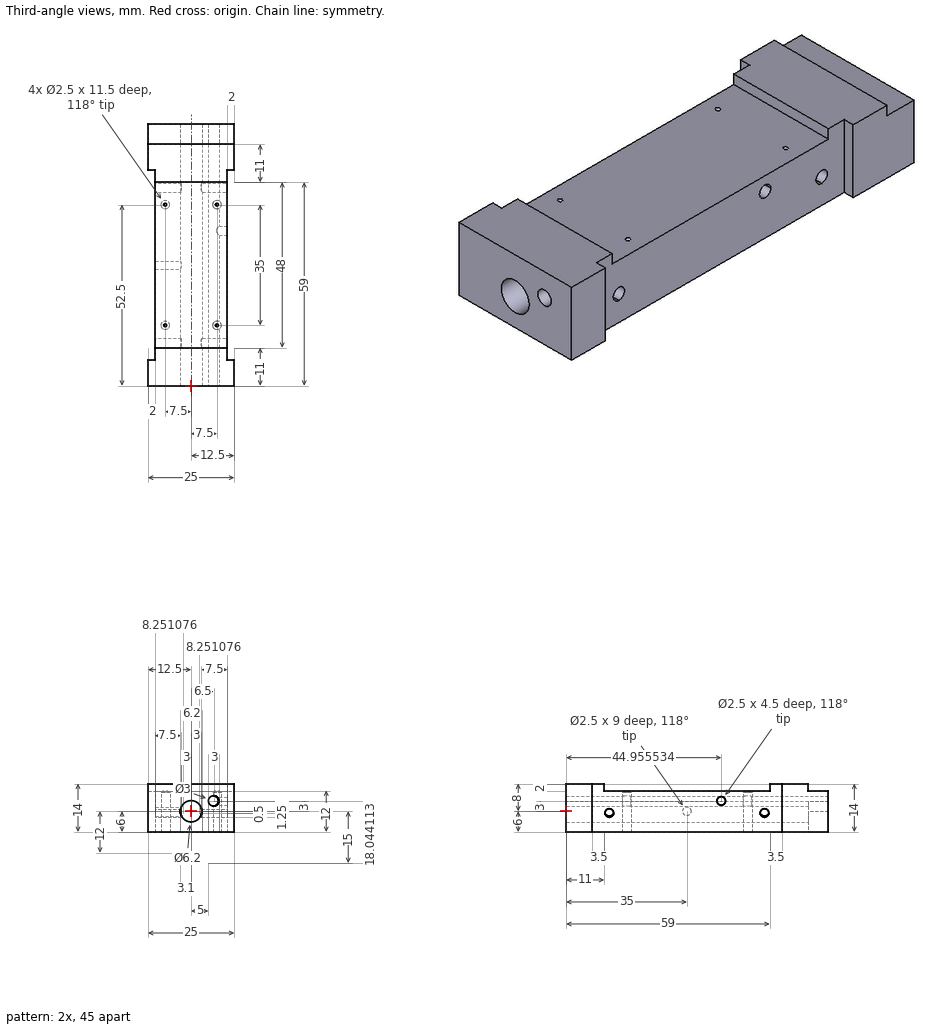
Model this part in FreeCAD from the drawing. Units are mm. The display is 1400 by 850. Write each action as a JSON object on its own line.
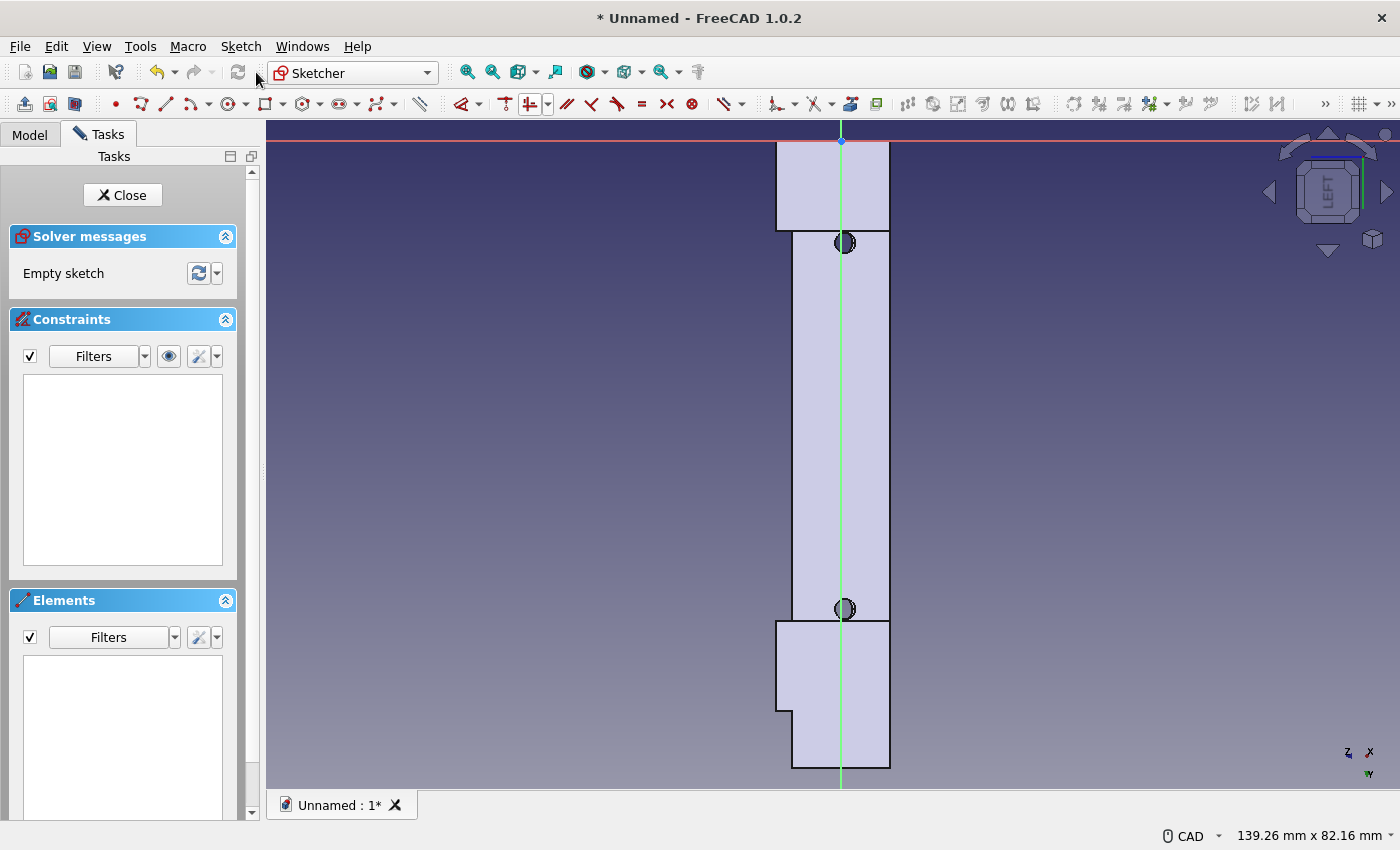
{"action": "scroll", "coordinate": [455, 721], "scroll_direction": "down", "scroll_amount": 1}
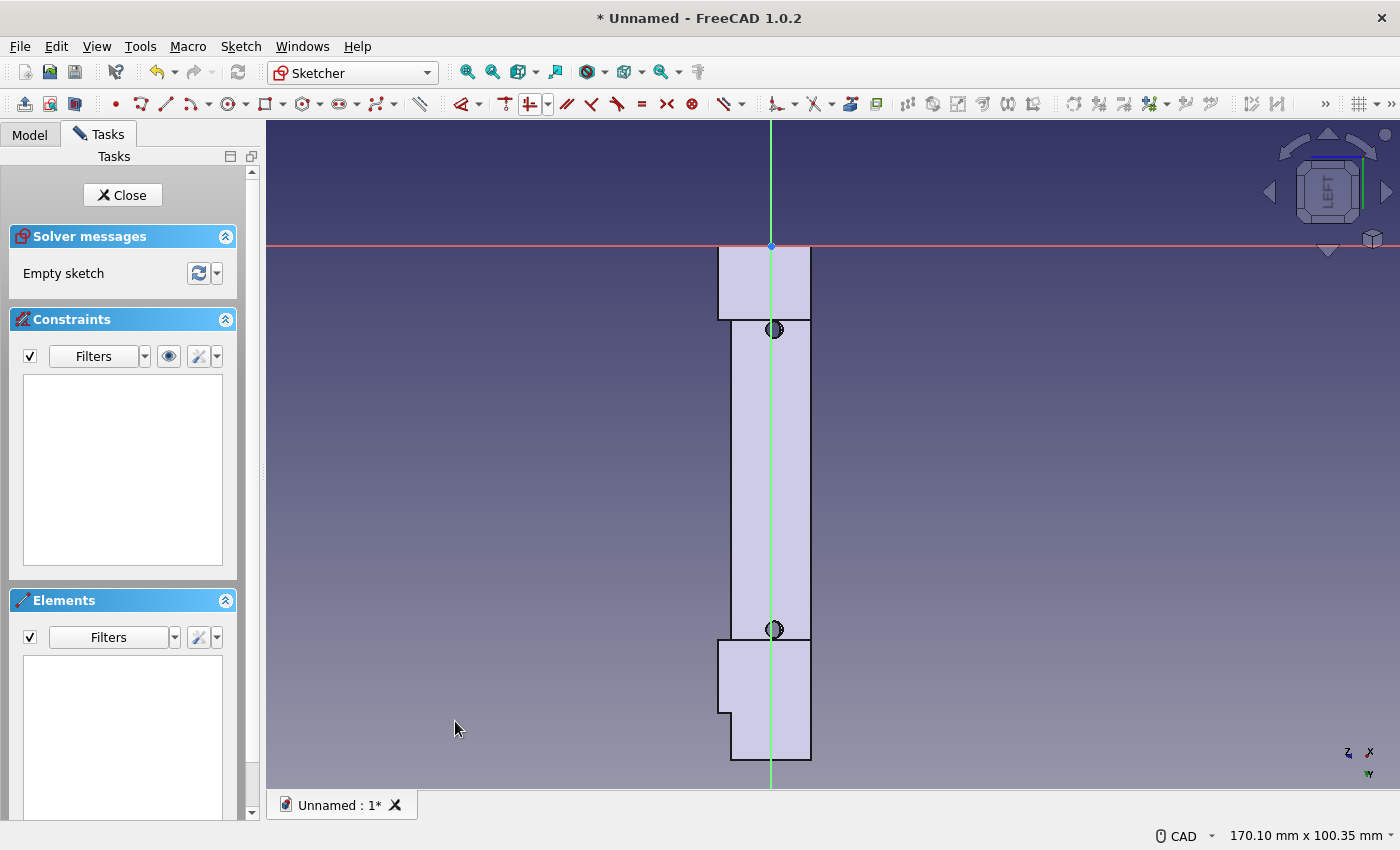
{"action": "left_click", "coordinate": [264, 104]}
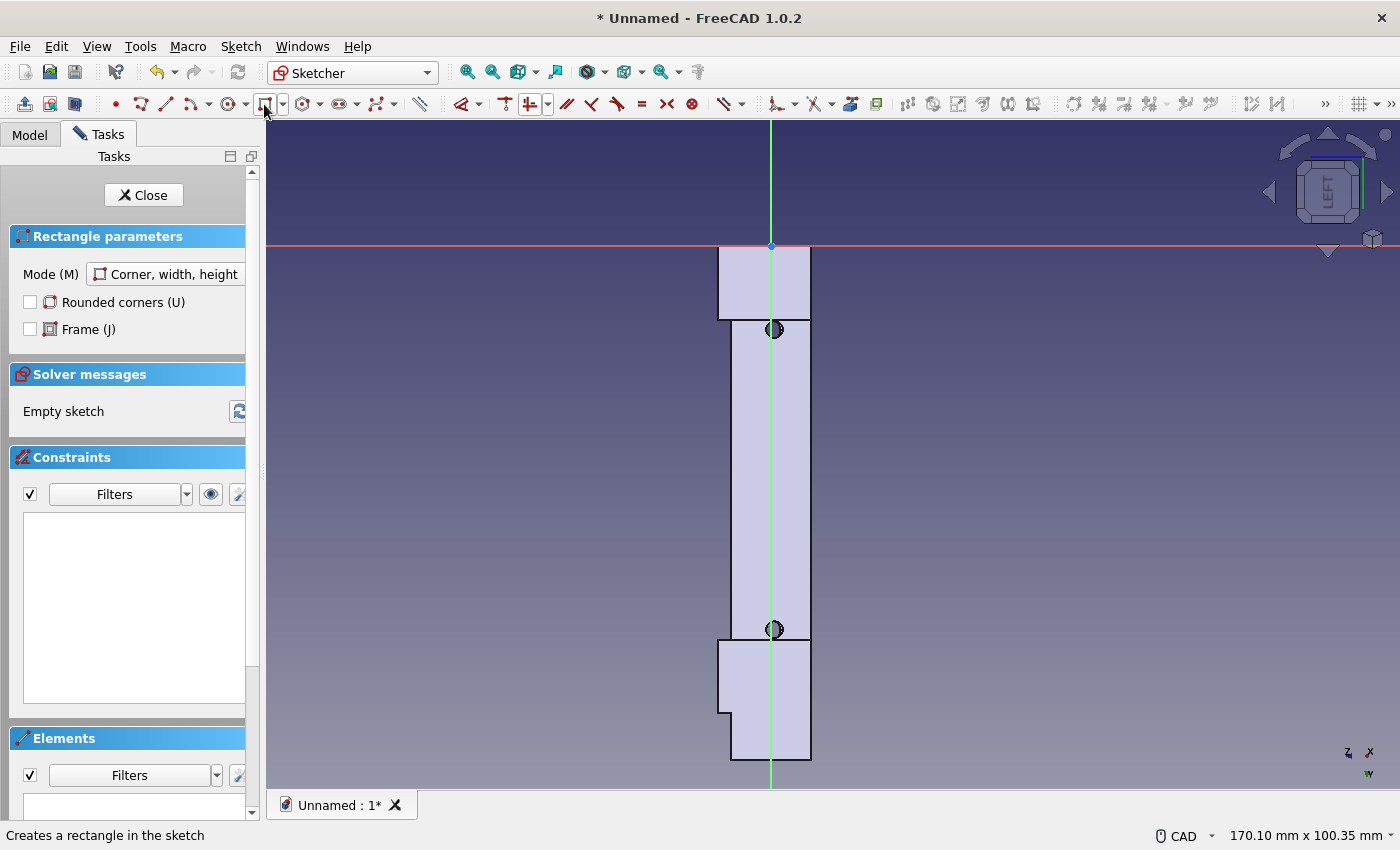
{"action": "left_click", "coordinate": [718, 640]}
{"action": "left_click", "coordinate": [811, 663]}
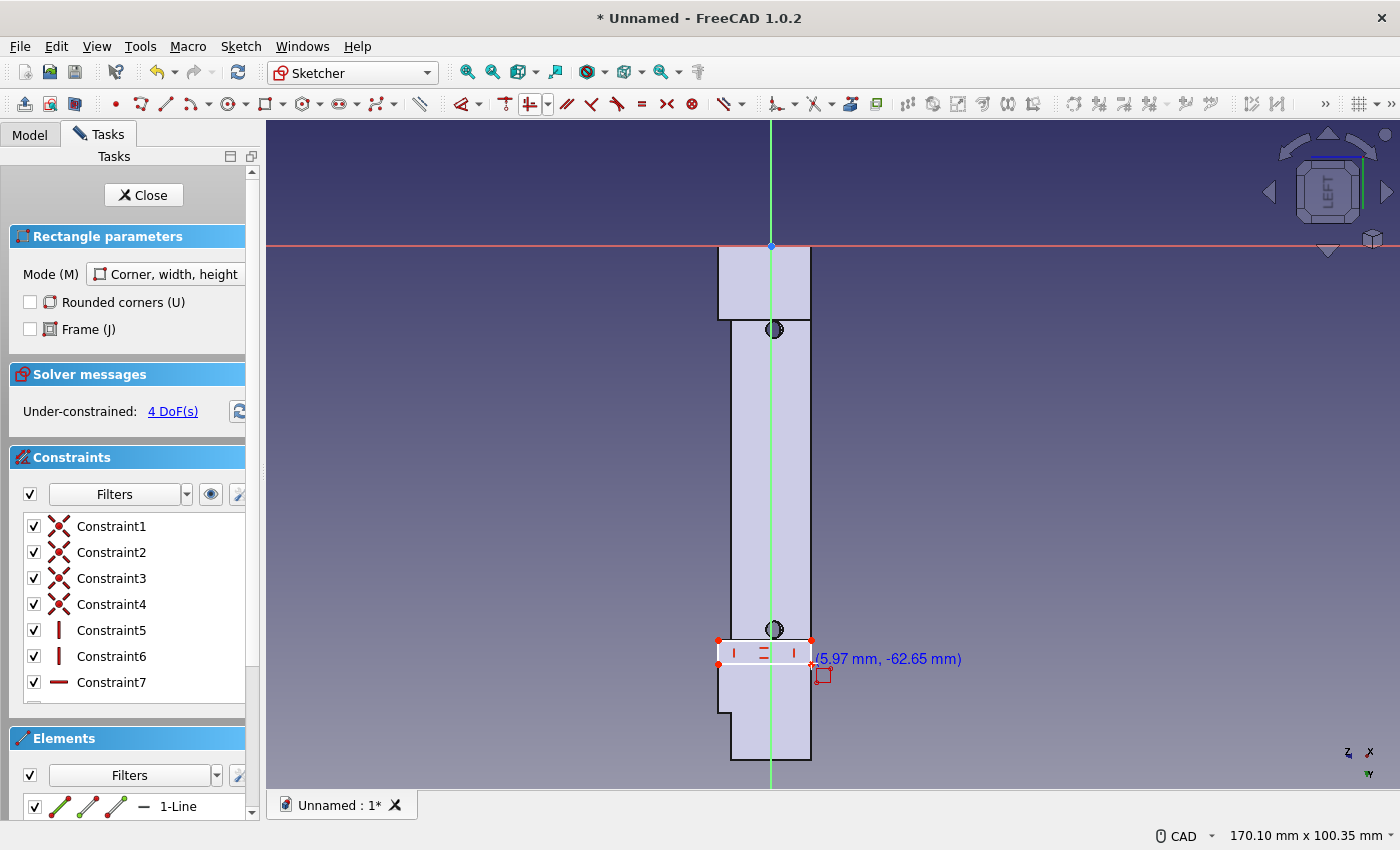
{"action": "left_click", "coordinate": [718, 296]}
{"action": "left_click", "coordinate": [811, 320]}
{"action": "key", "text": "Escape"}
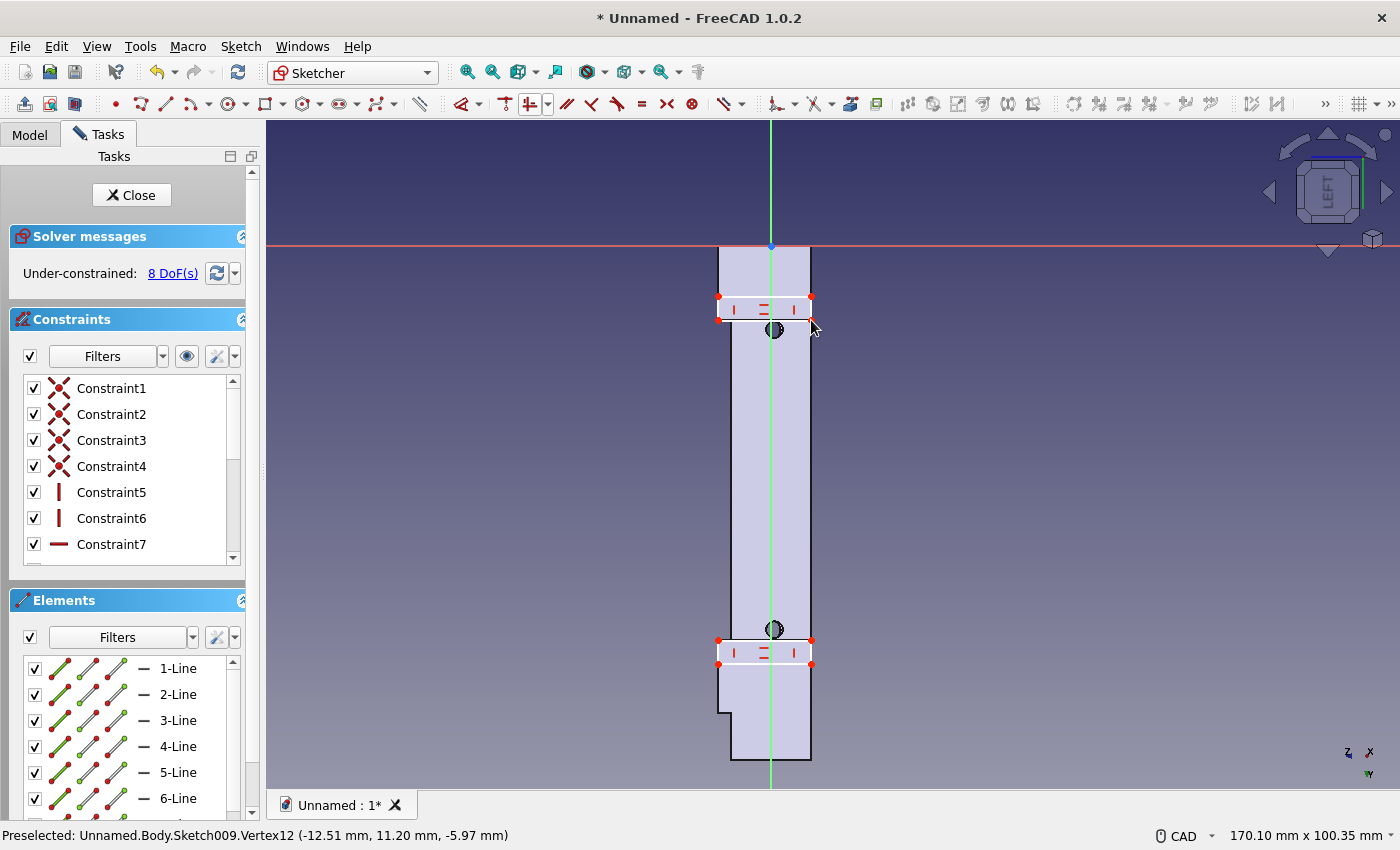
{"action": "left_click", "coordinate": [460, 104]}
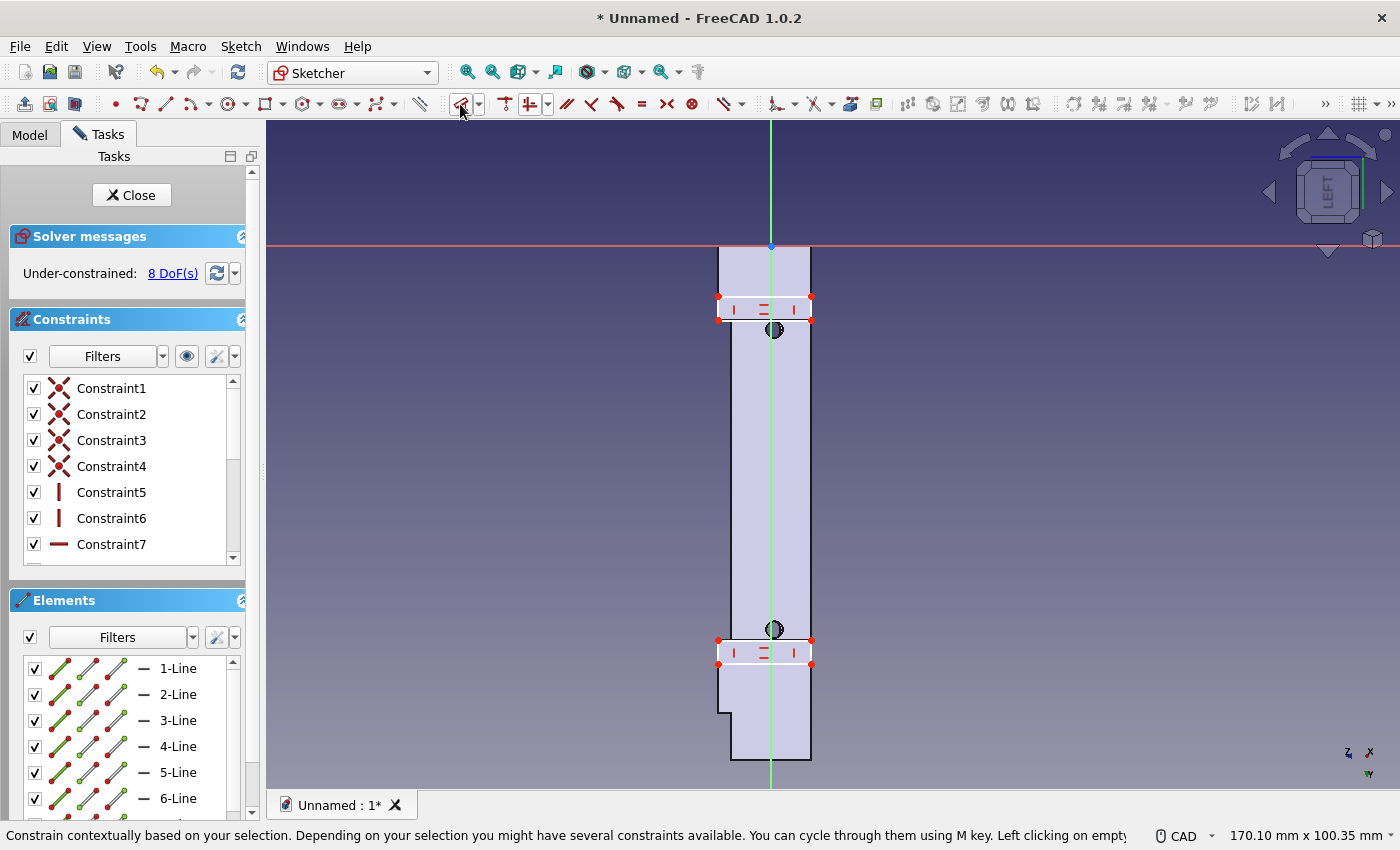
{"action": "left_click", "coordinate": [746, 664]}
{"action": "left_click", "coordinate": [743, 698]}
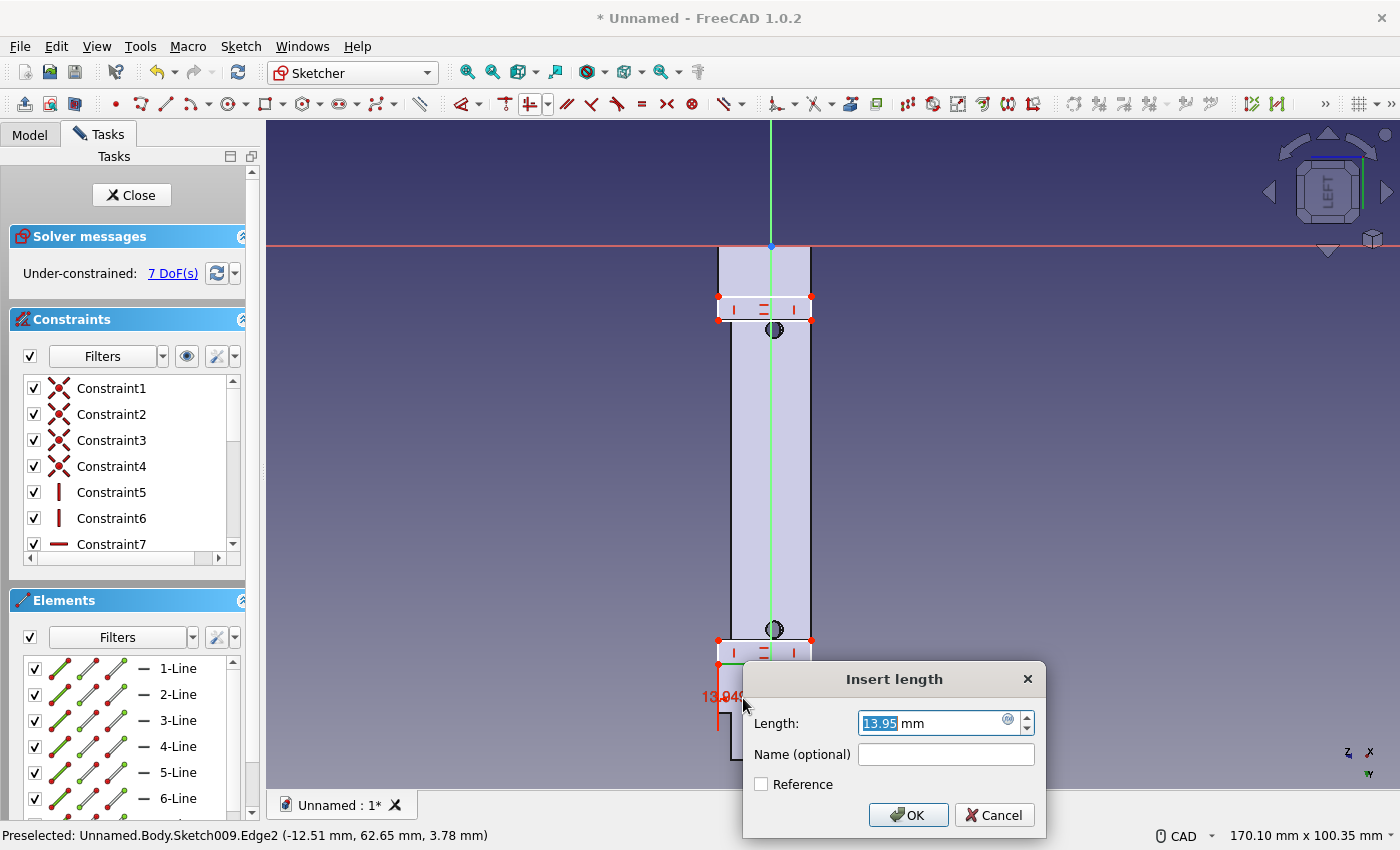
{"action": "type", "text": "14"}
{"action": "key", "text": "Return"}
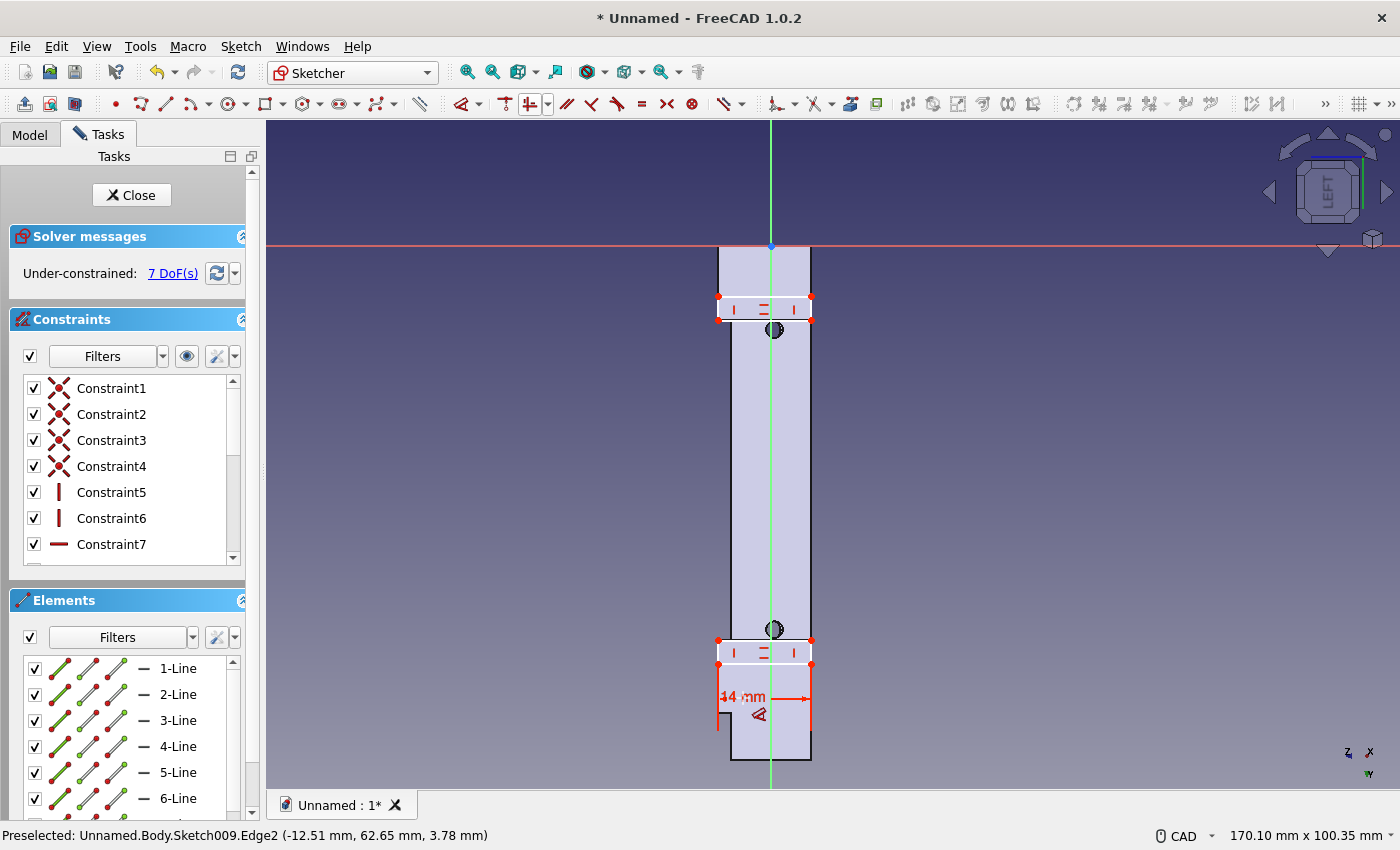
{"action": "left_click", "coordinate": [746, 321]}
{"action": "left_click", "coordinate": [743, 355]}